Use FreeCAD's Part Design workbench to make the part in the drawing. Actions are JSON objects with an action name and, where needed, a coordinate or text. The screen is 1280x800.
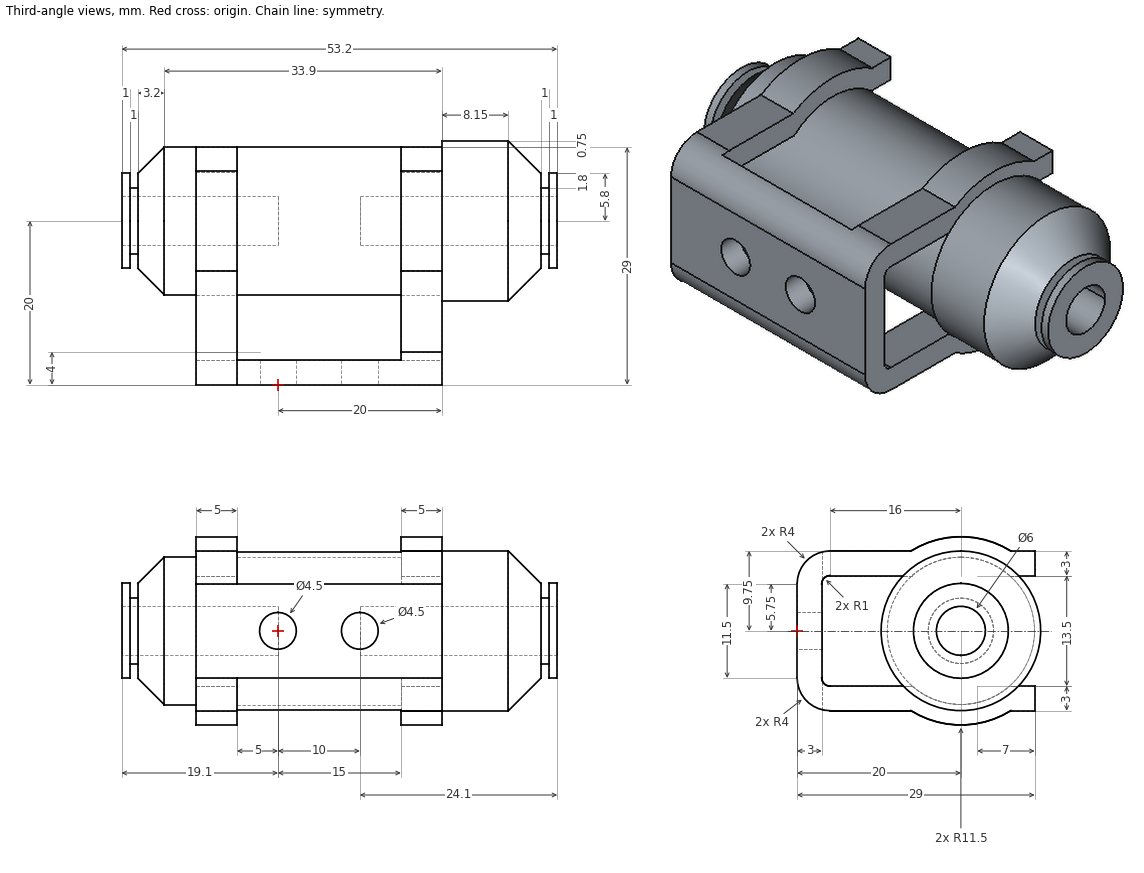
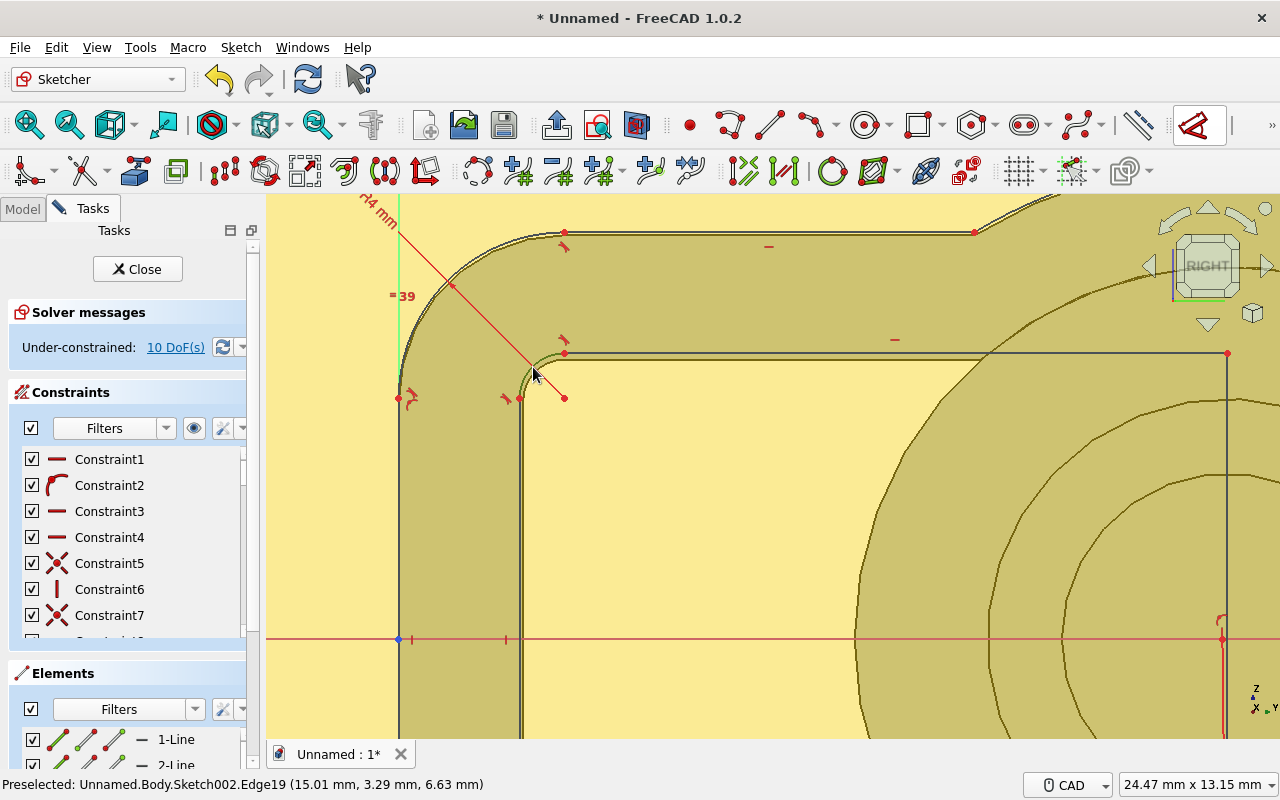
{"action": "left_click", "coordinate": [1220, 126]}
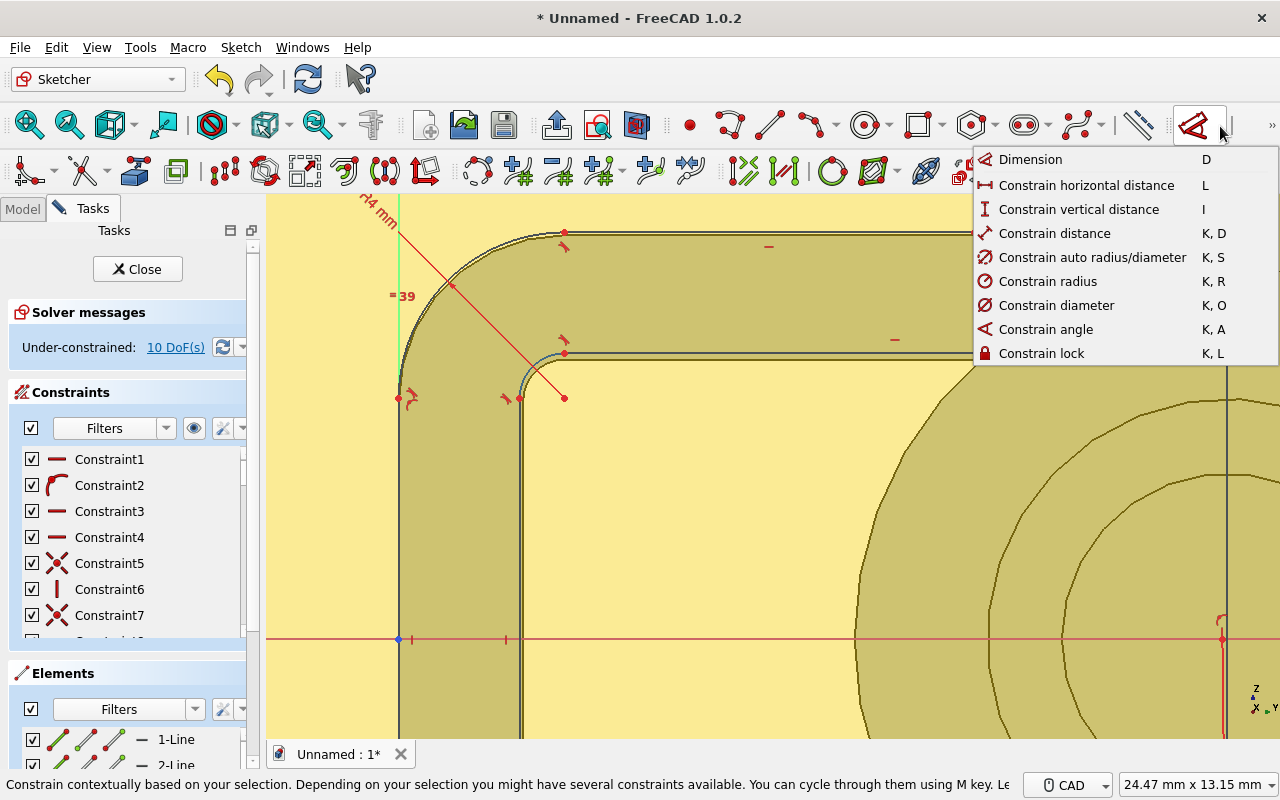
{"action": "left_click", "coordinate": [1126, 281]}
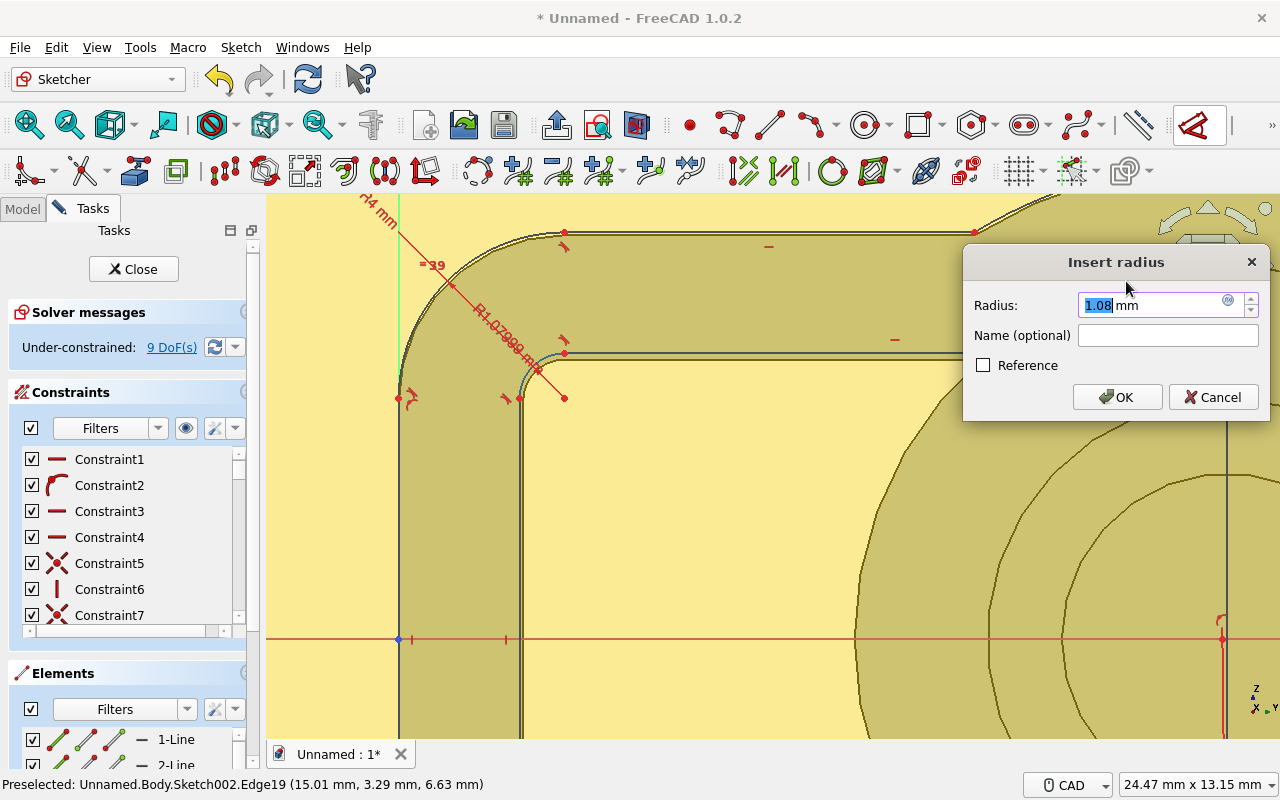
{"action": "type", "text": "1"}
{"action": "key", "text": "Return"}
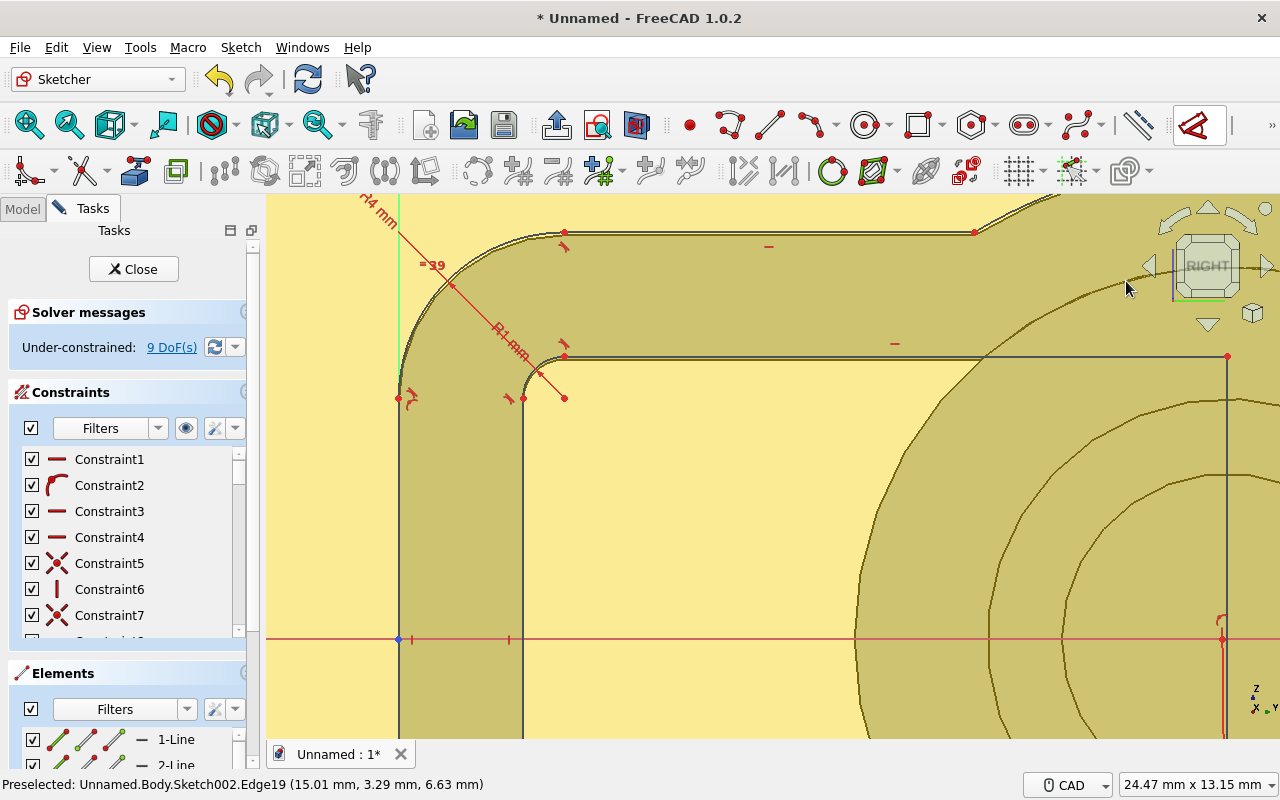
{"action": "scroll", "coordinate": [533, 366], "scroll_direction": "down", "scroll_amount": 5}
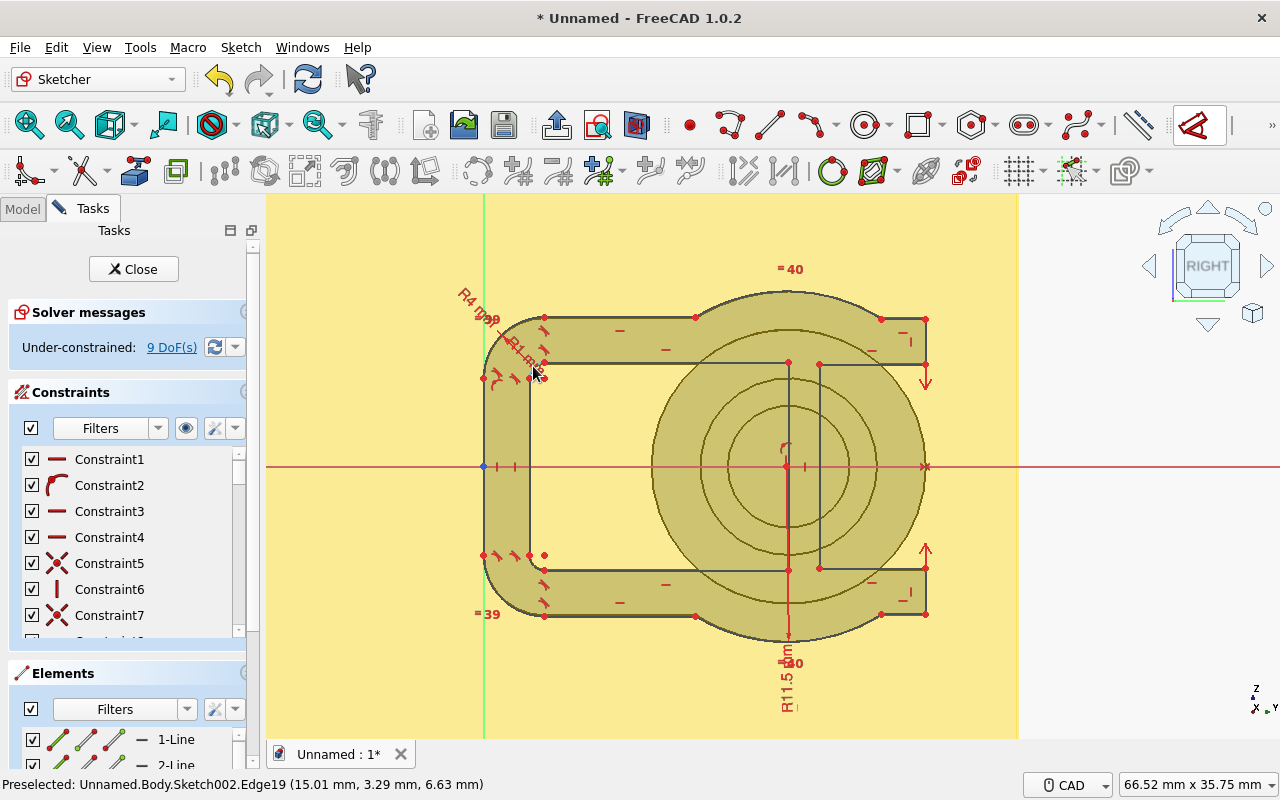
{"action": "left_click", "coordinate": [926, 601]}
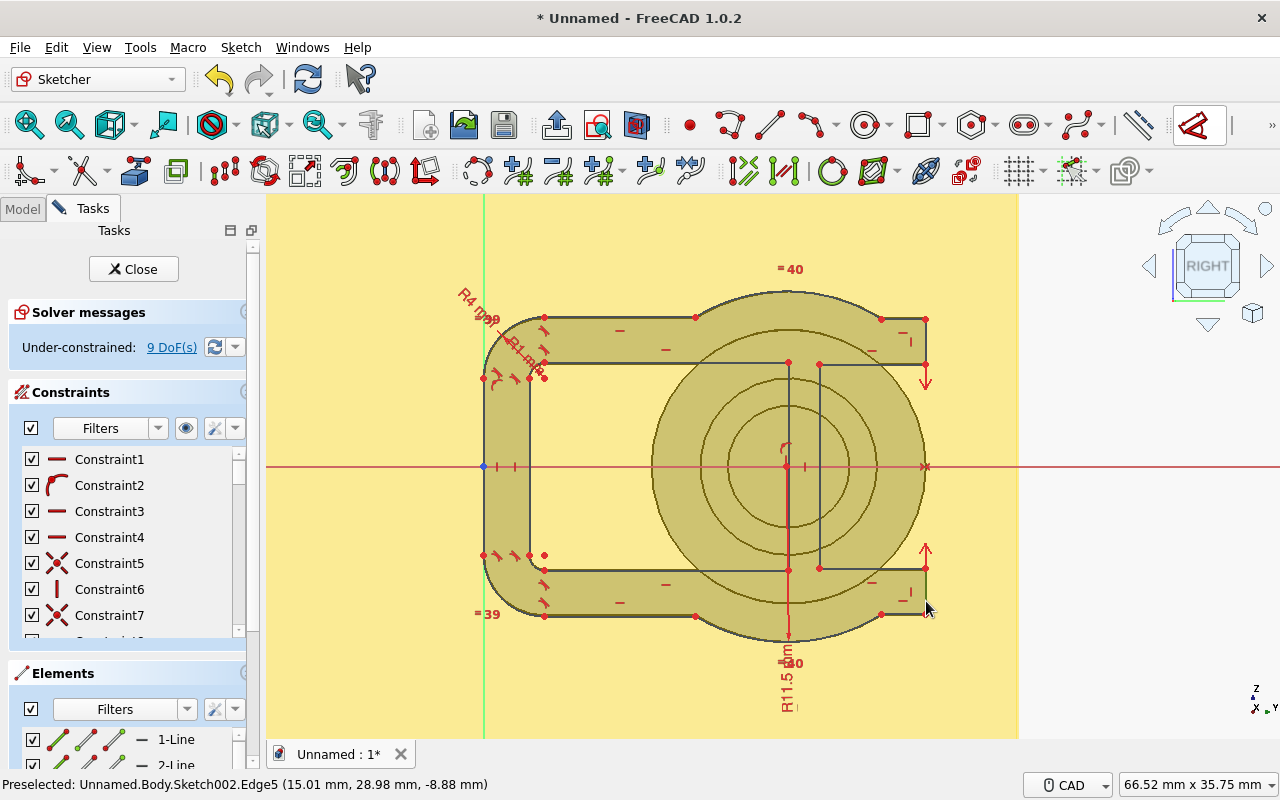
{"action": "left_click", "coordinate": [1220, 126]}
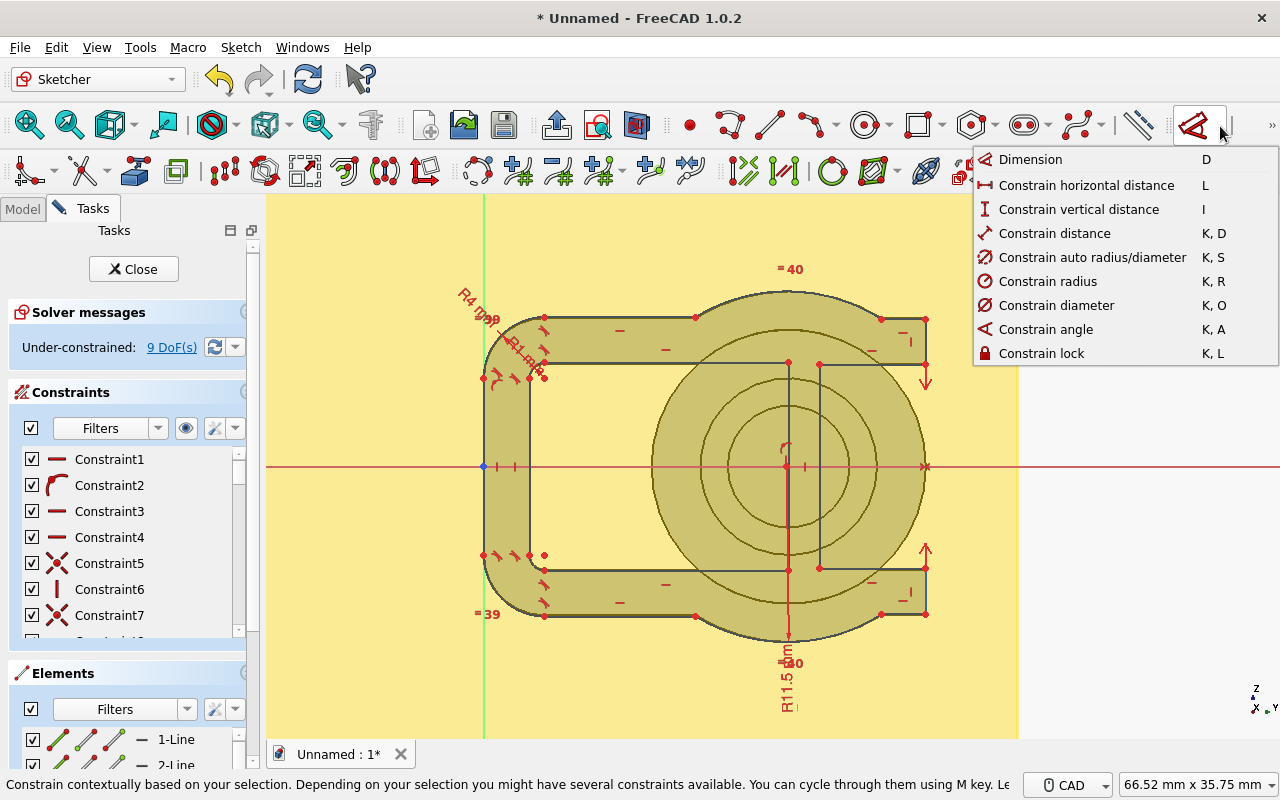
{"action": "left_click", "coordinate": [1126, 209]}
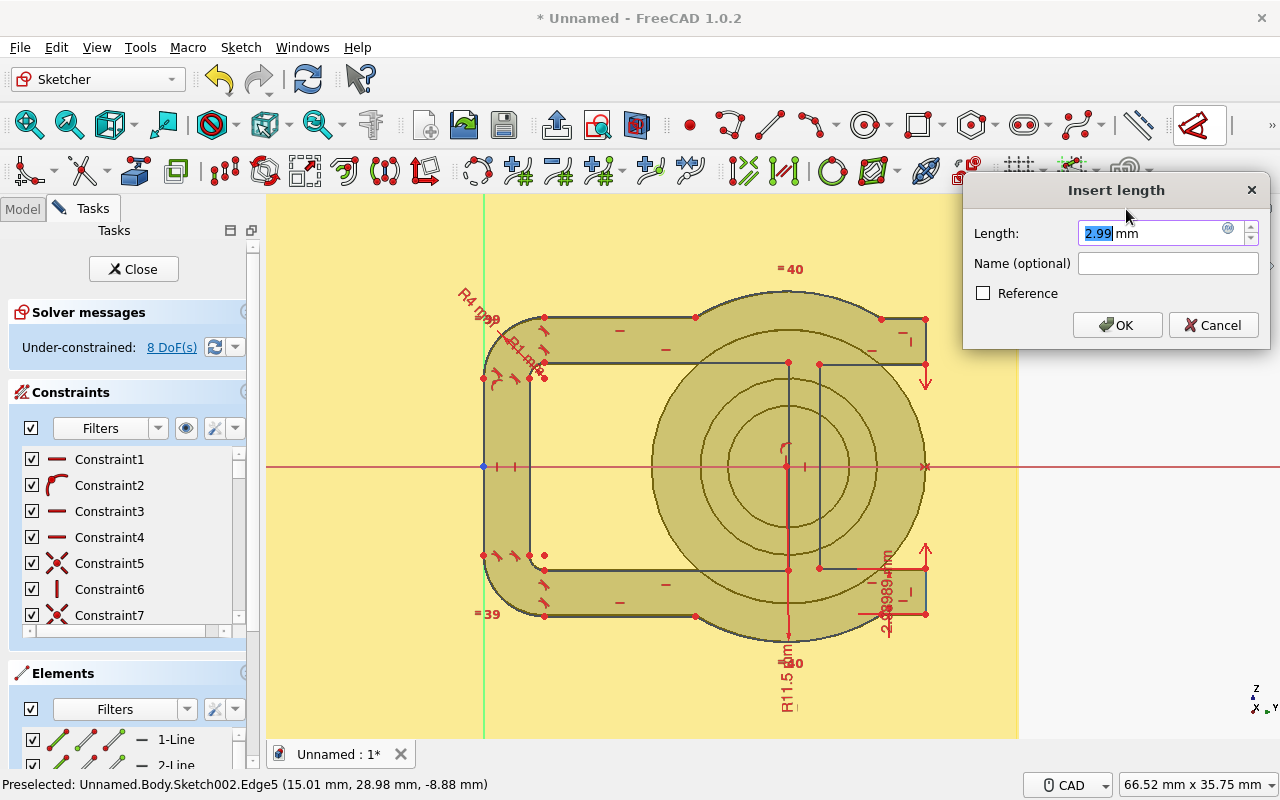
{"action": "type", "text": "3"}
{"action": "key", "text": "Return"}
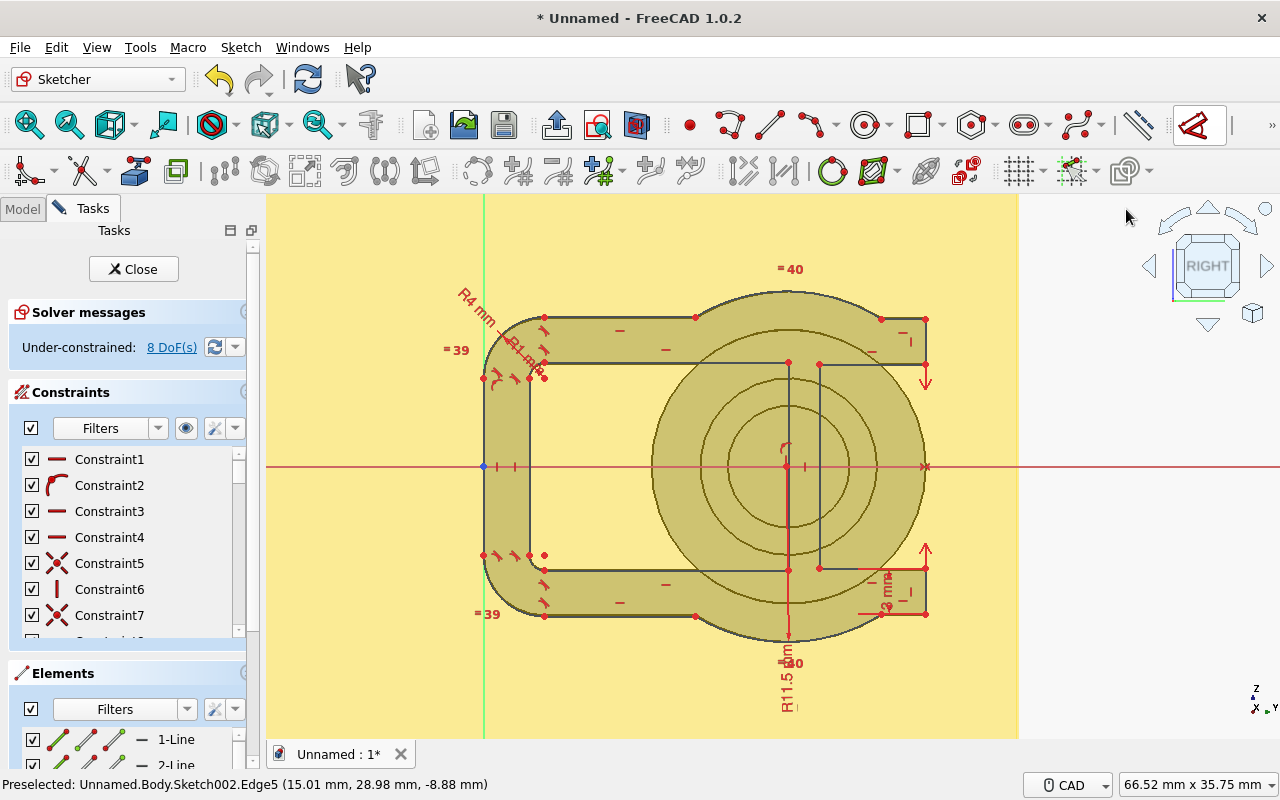
{"action": "left_click", "coordinate": [894, 569]}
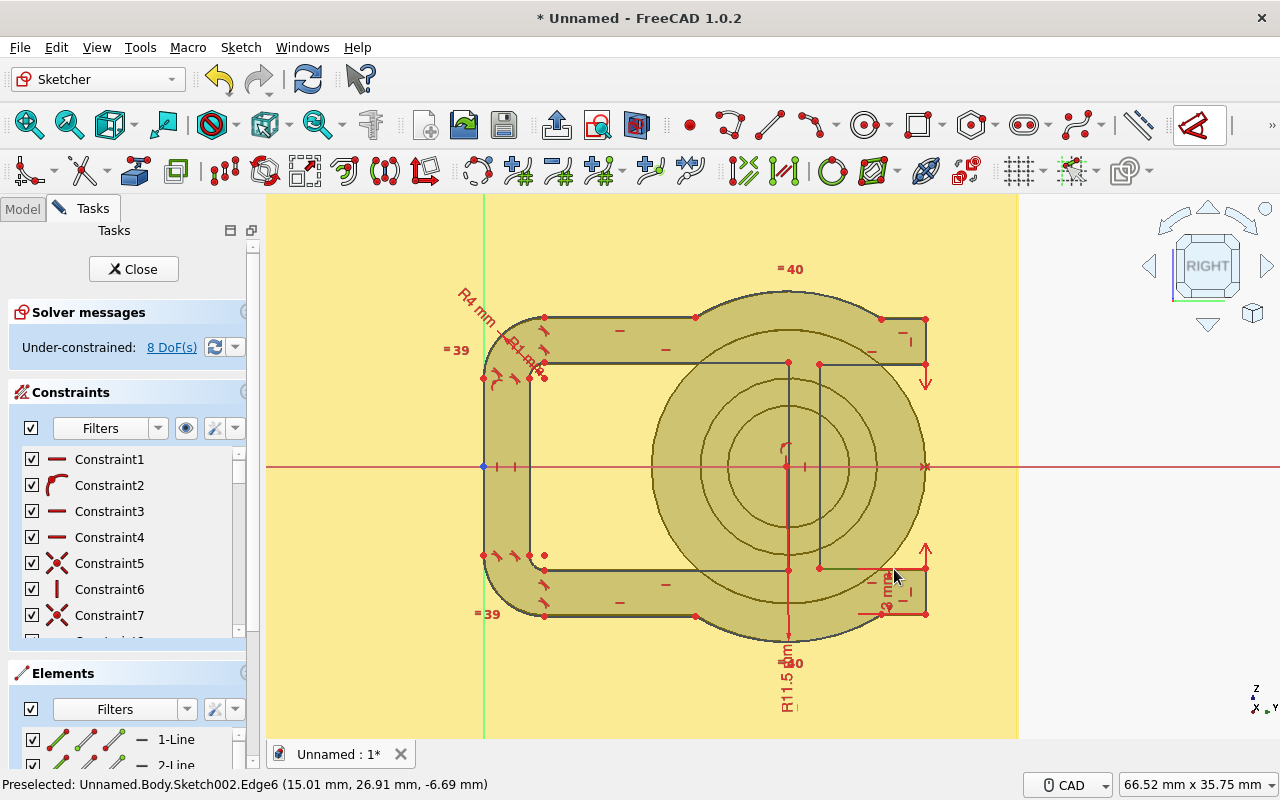
{"action": "left_click", "coordinate": [1220, 126]}